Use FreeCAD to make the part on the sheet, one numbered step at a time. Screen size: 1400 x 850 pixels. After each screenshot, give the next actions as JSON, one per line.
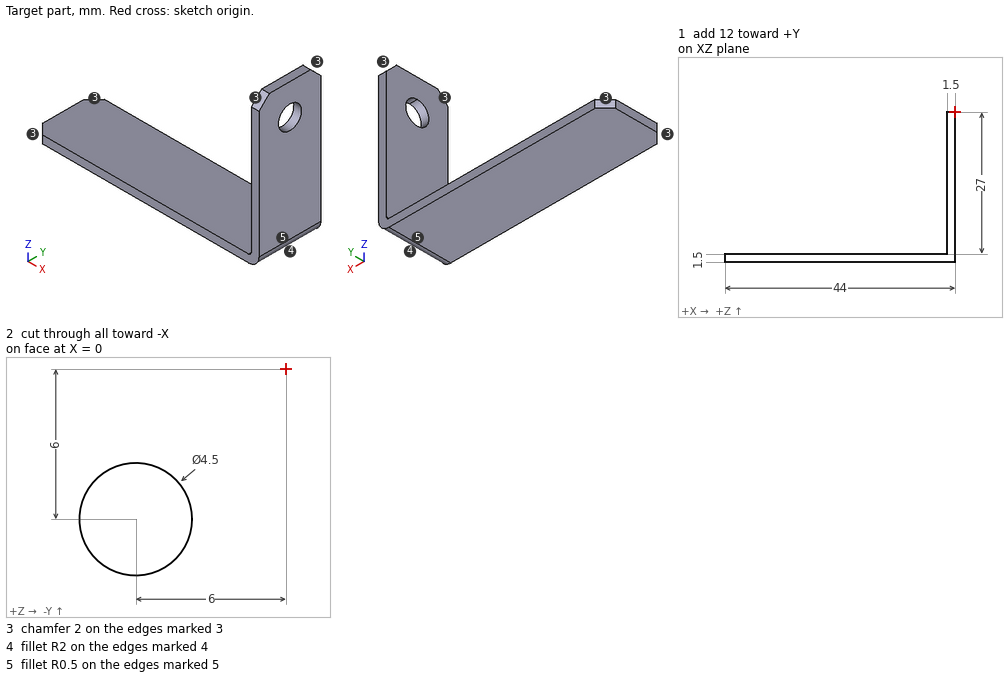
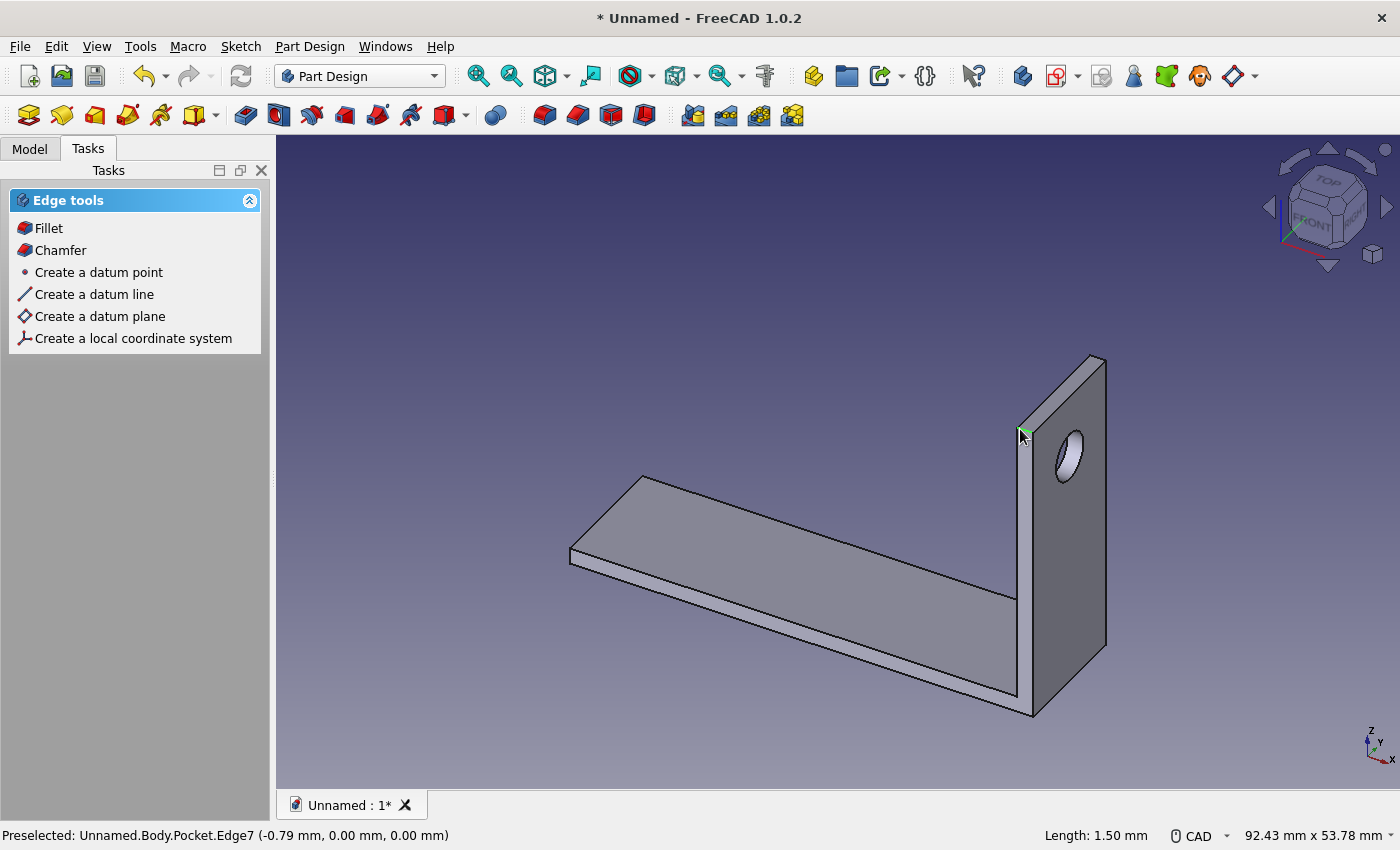
{"action": "scroll", "coordinate": [643, 483], "scroll_direction": "up", "scroll_amount": 4}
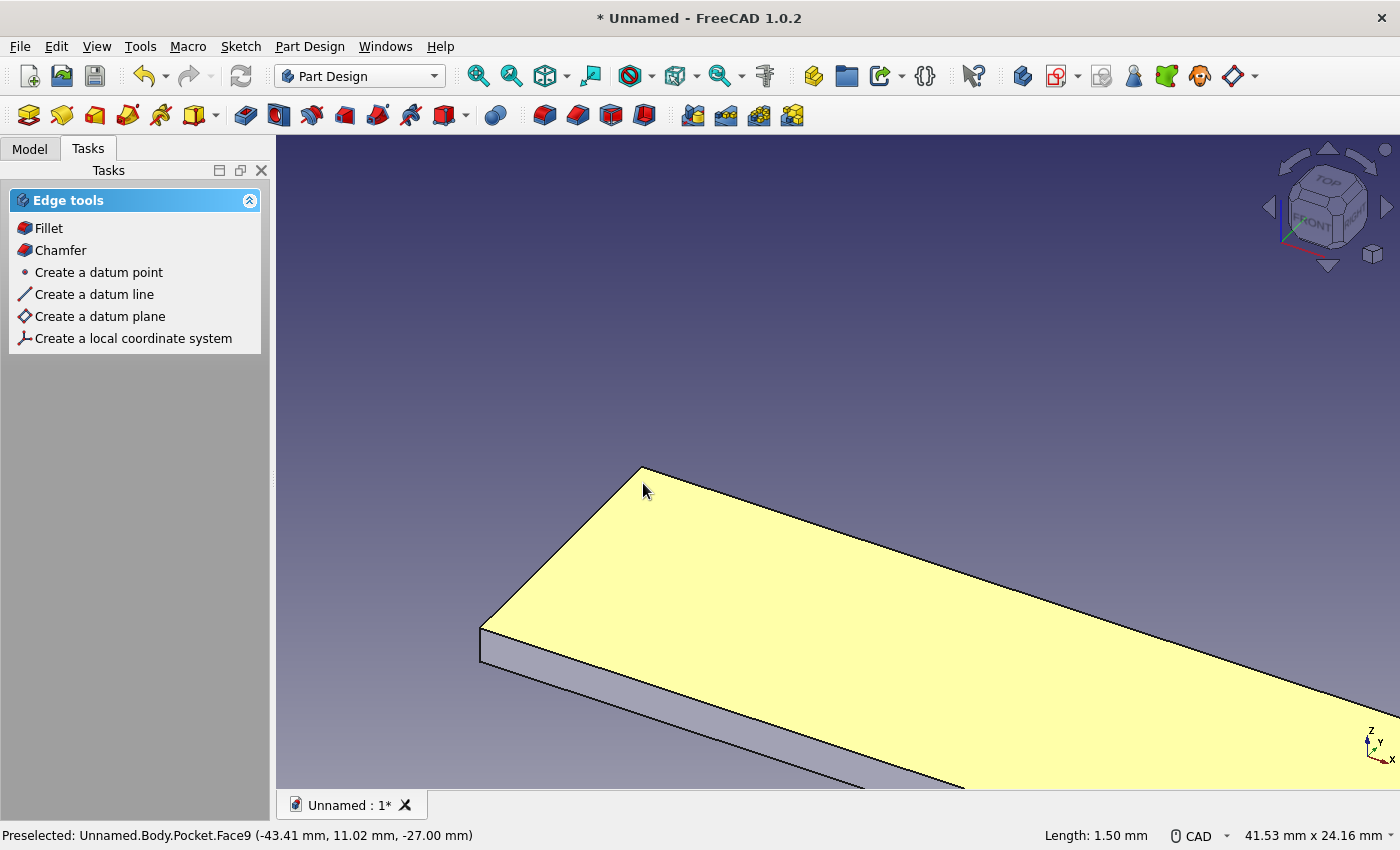
{"action": "left_click", "coordinate": [479, 76]}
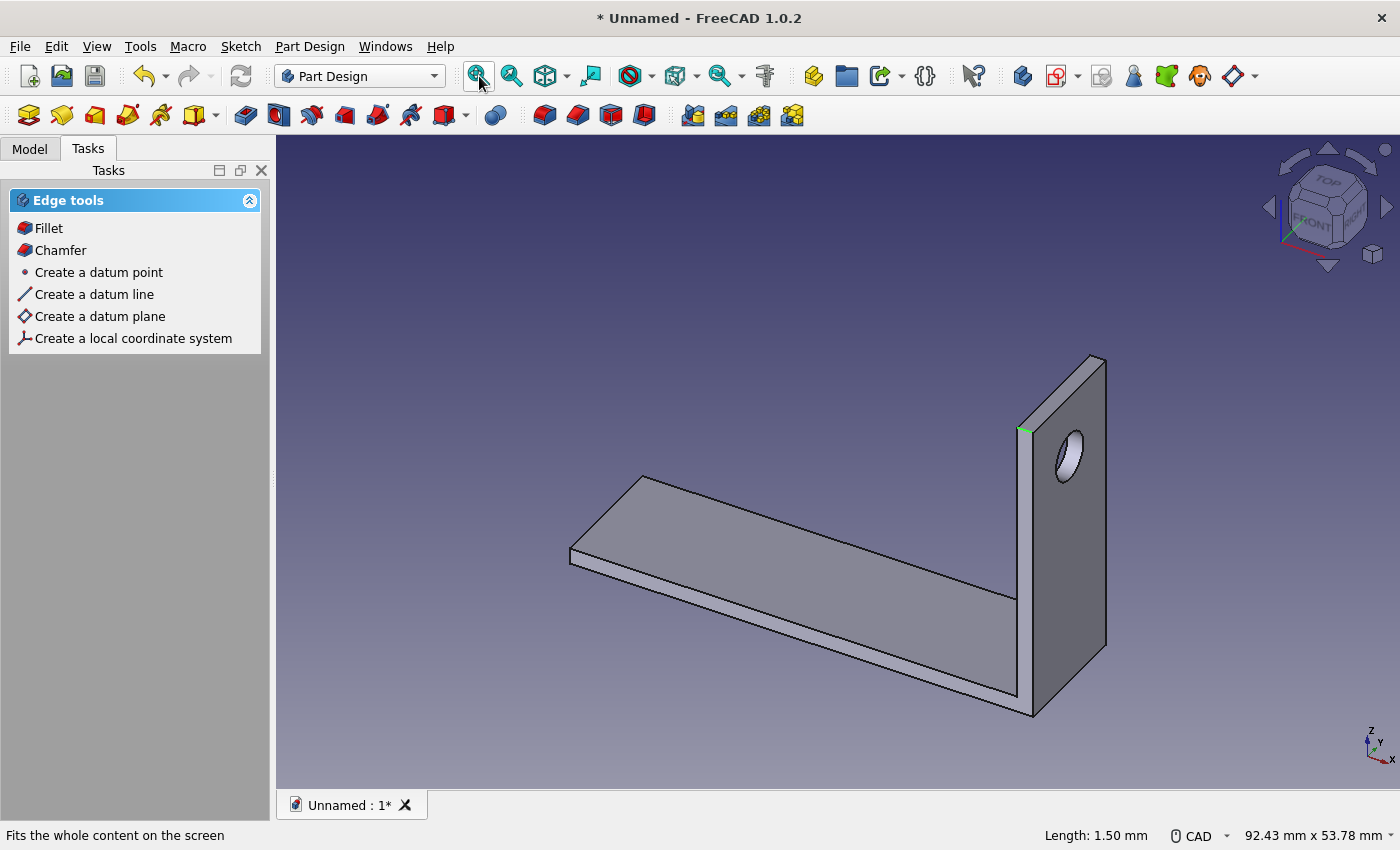
{"action": "key", "text": "0"}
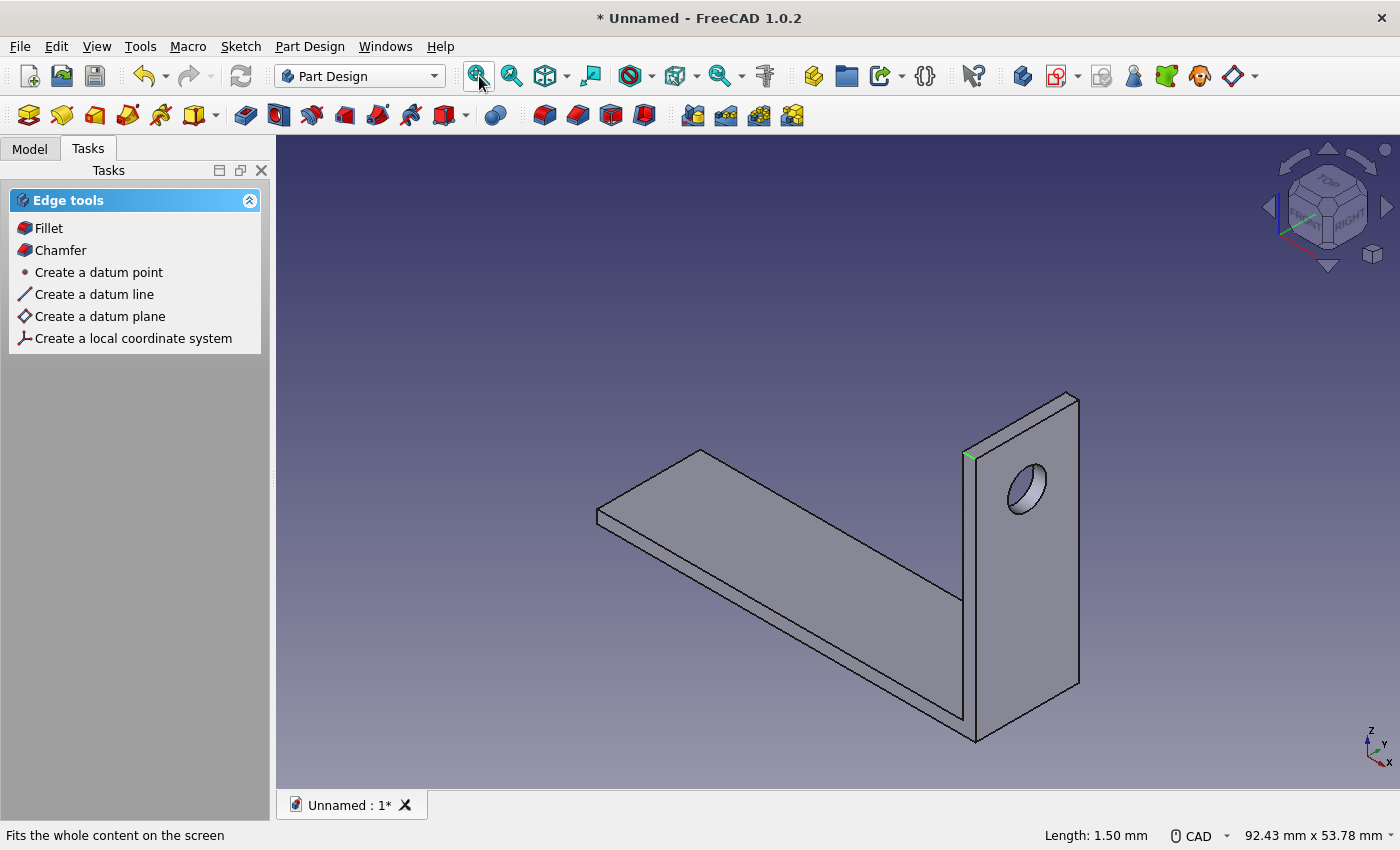
{"action": "scroll", "coordinate": [700, 456], "scroll_direction": "up", "scroll_amount": 4}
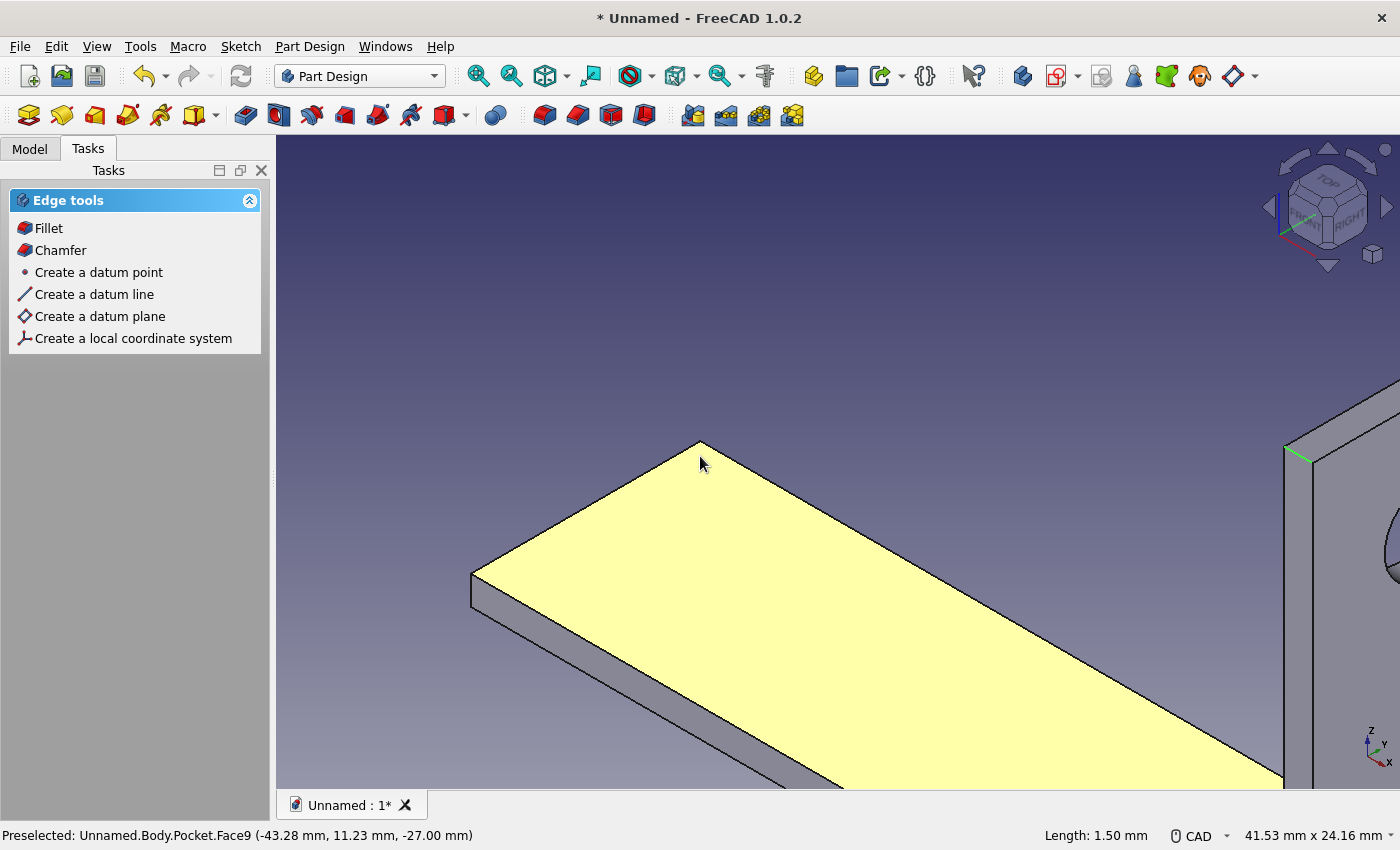
{"action": "left_click", "coordinate": [479, 76]}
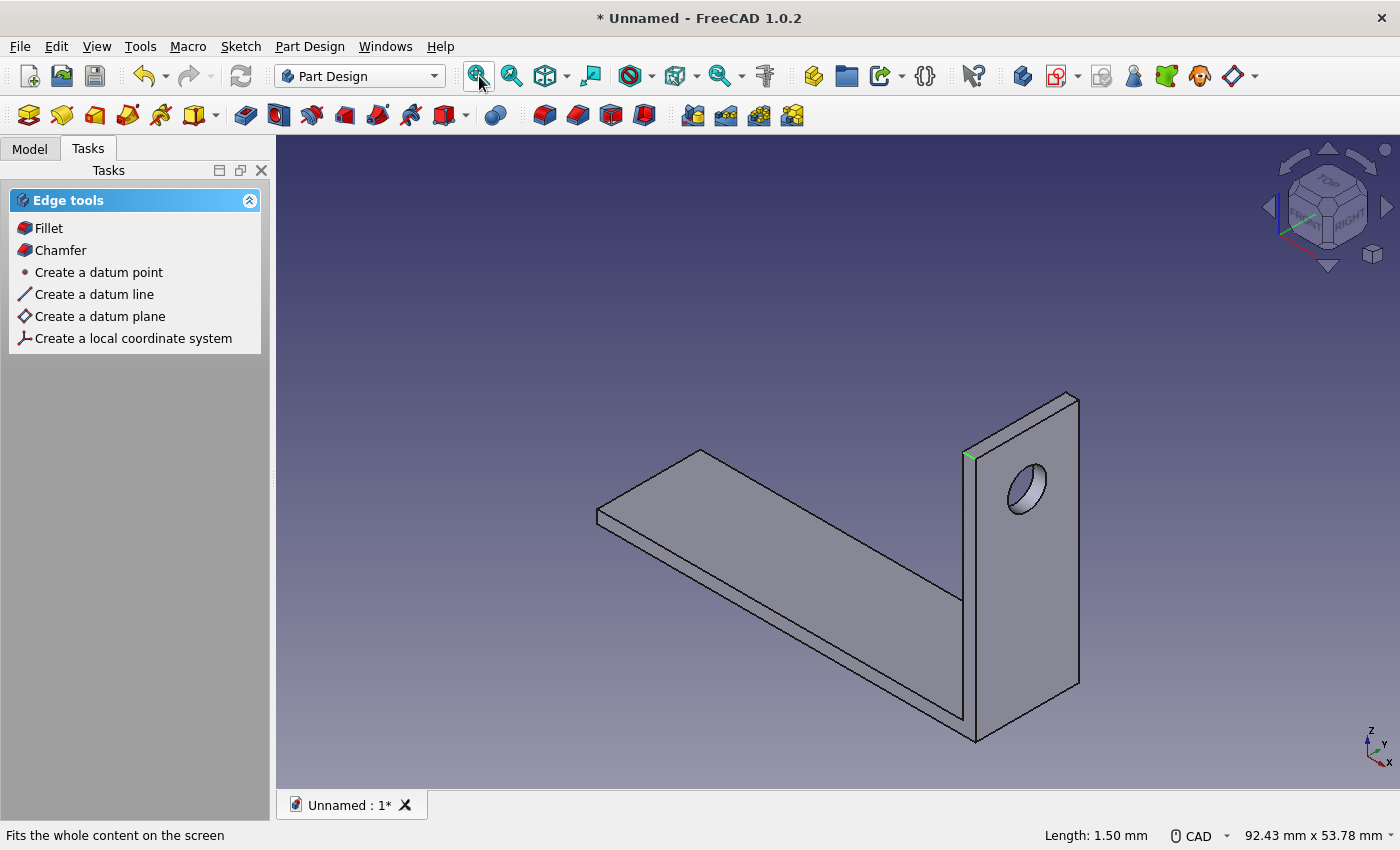
{"action": "key", "text": "2"}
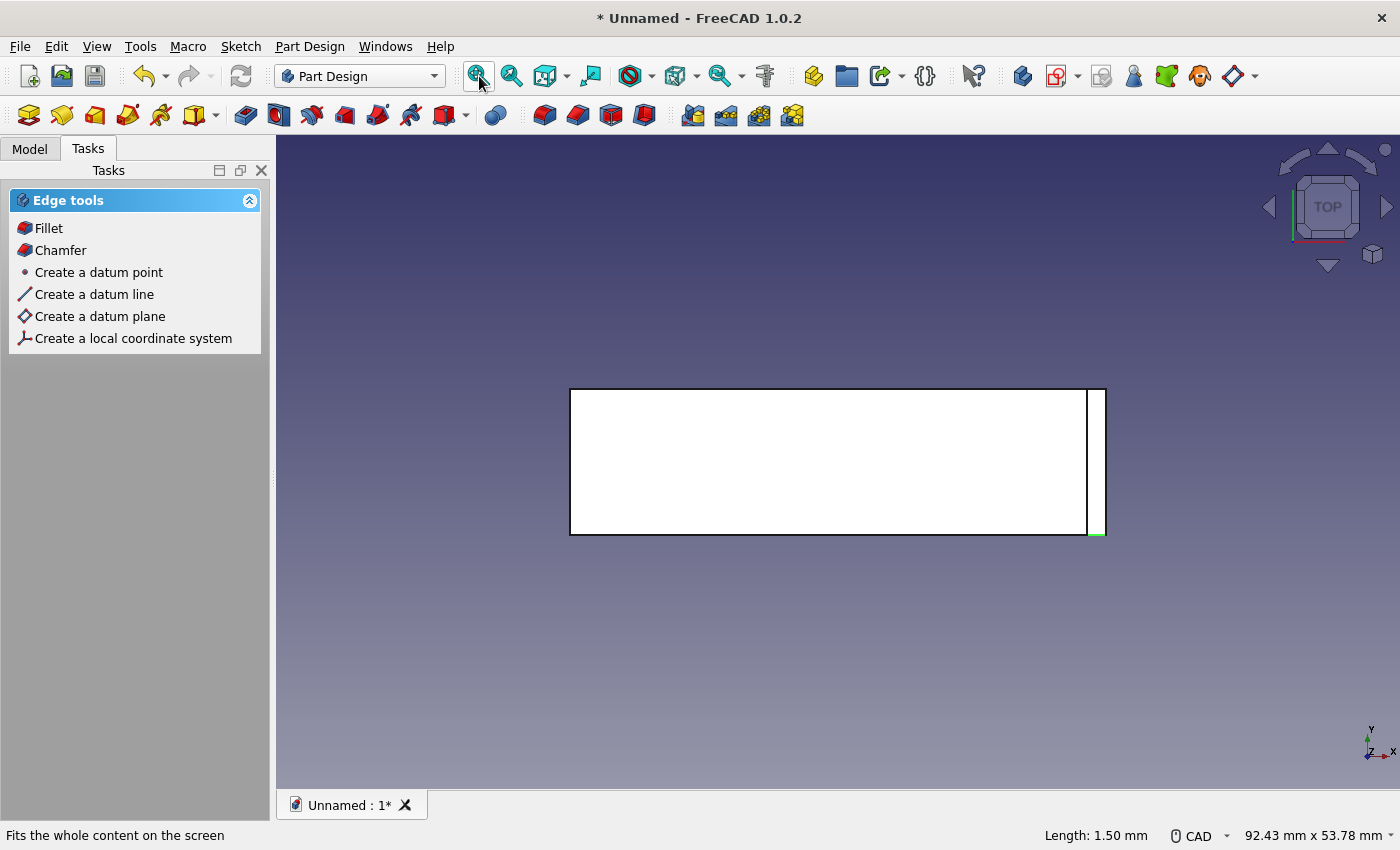
{"action": "left_click", "coordinate": [1096, 388], "text": "ctrl"}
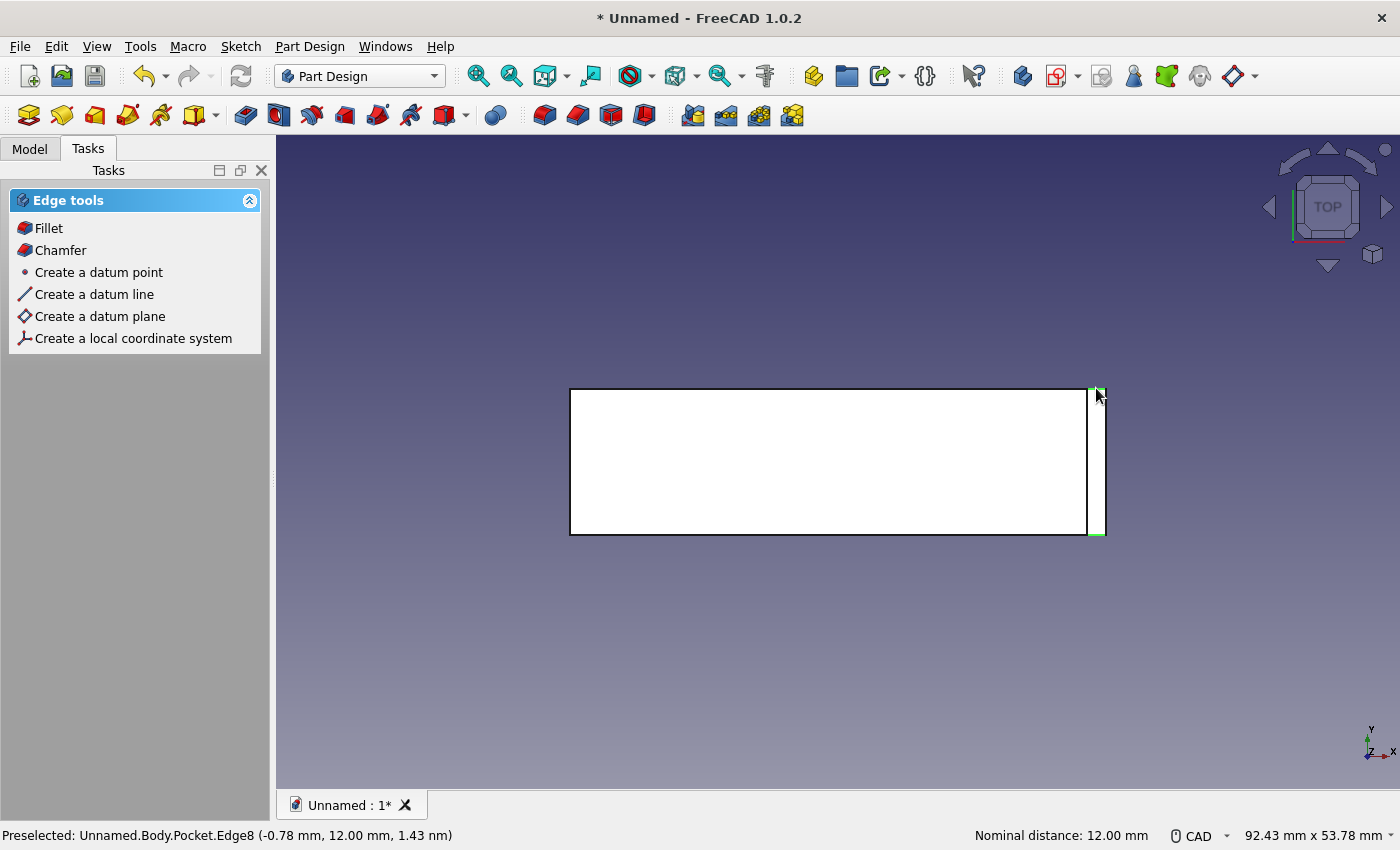
{"action": "scroll", "coordinate": [570, 388], "scroll_direction": "up", "scroll_amount": 4}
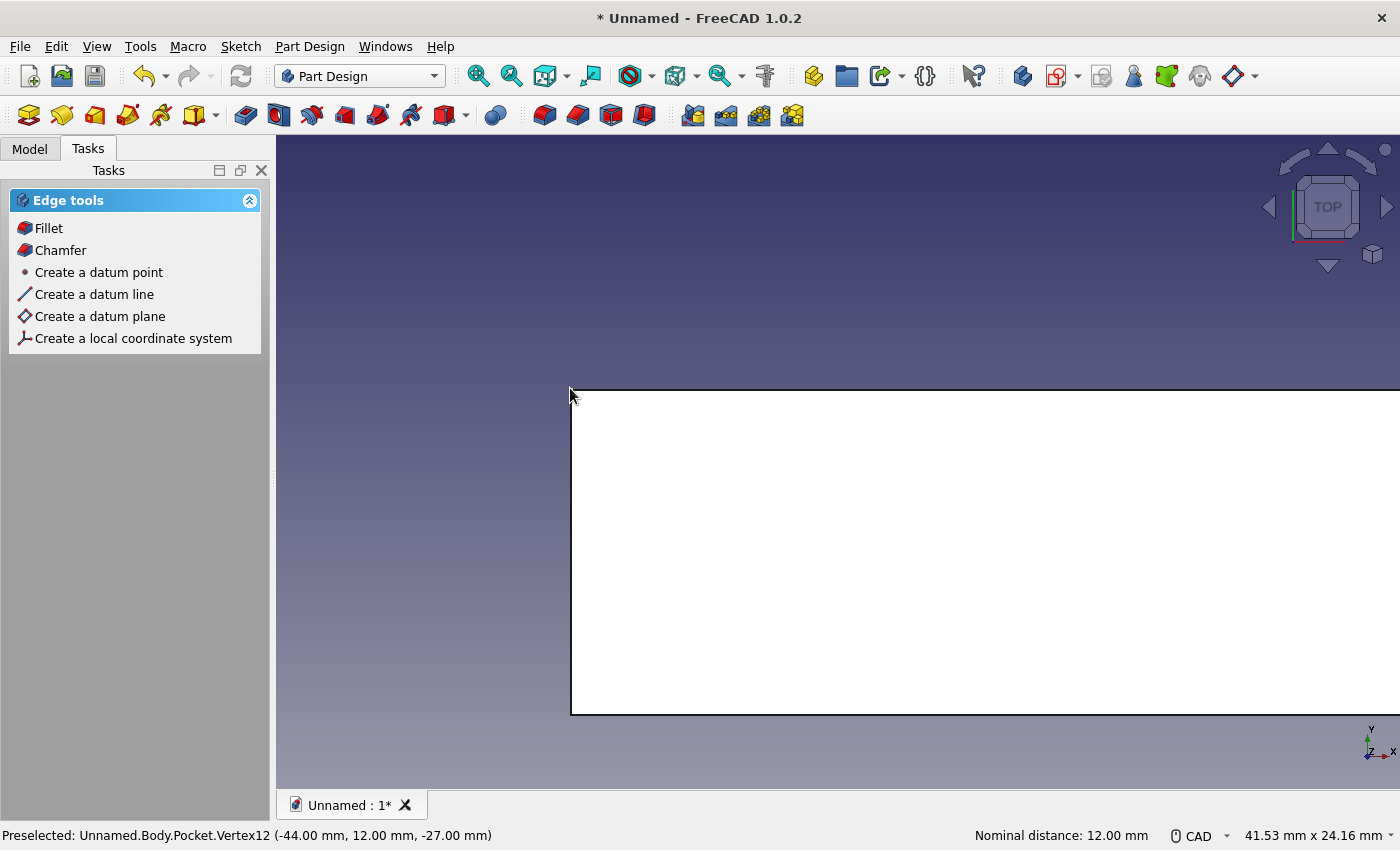
{"action": "key", "text": "v f"}